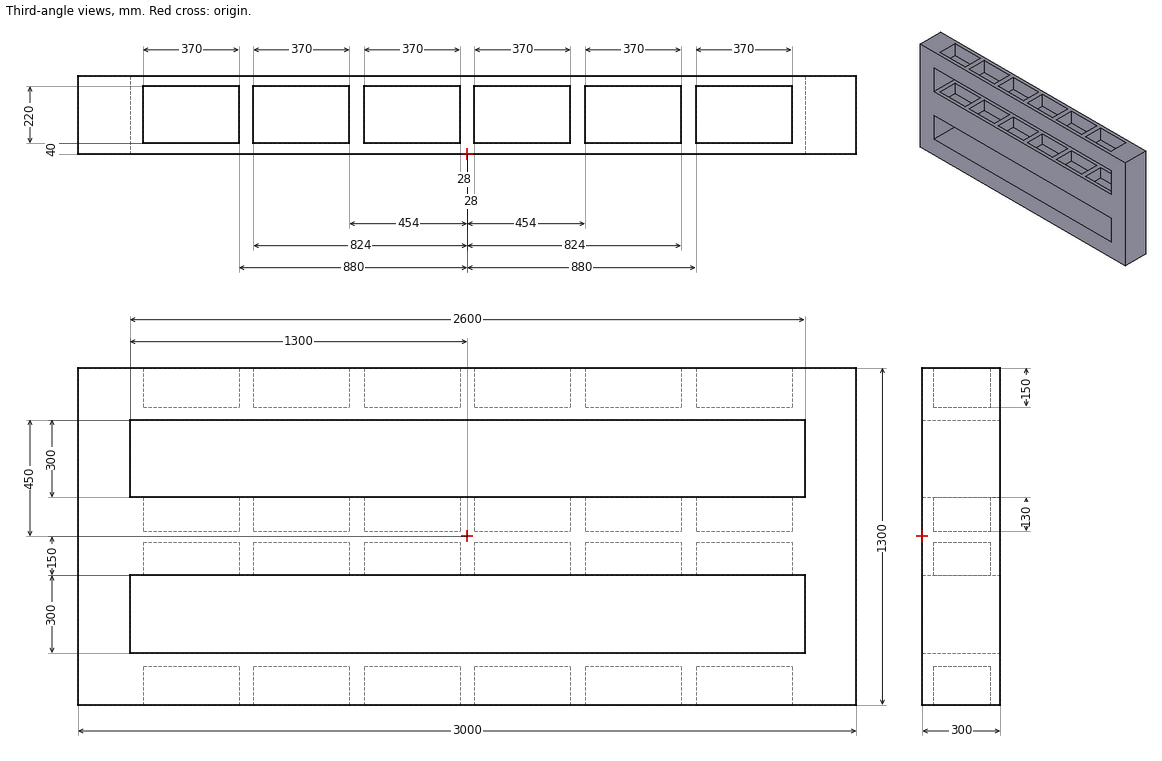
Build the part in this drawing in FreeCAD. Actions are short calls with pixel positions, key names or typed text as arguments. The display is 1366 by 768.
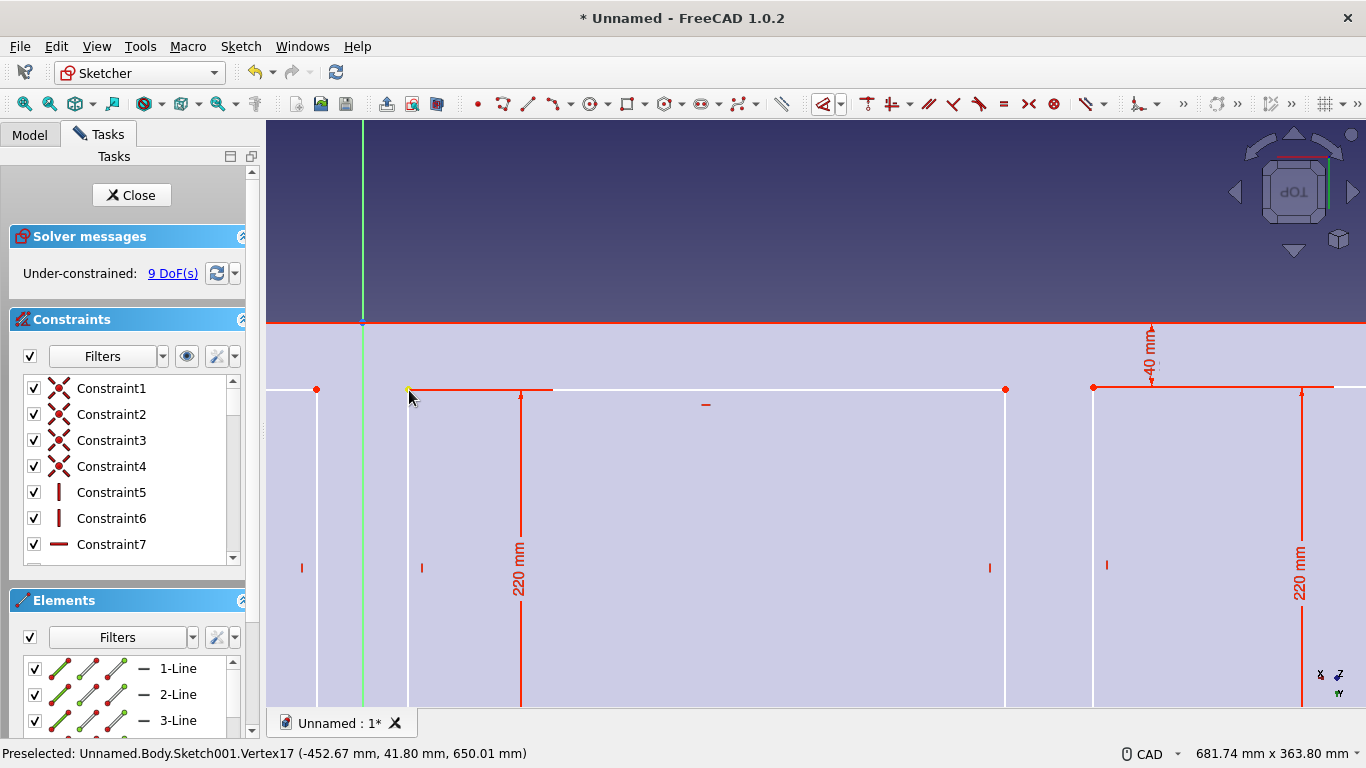
click(408, 390)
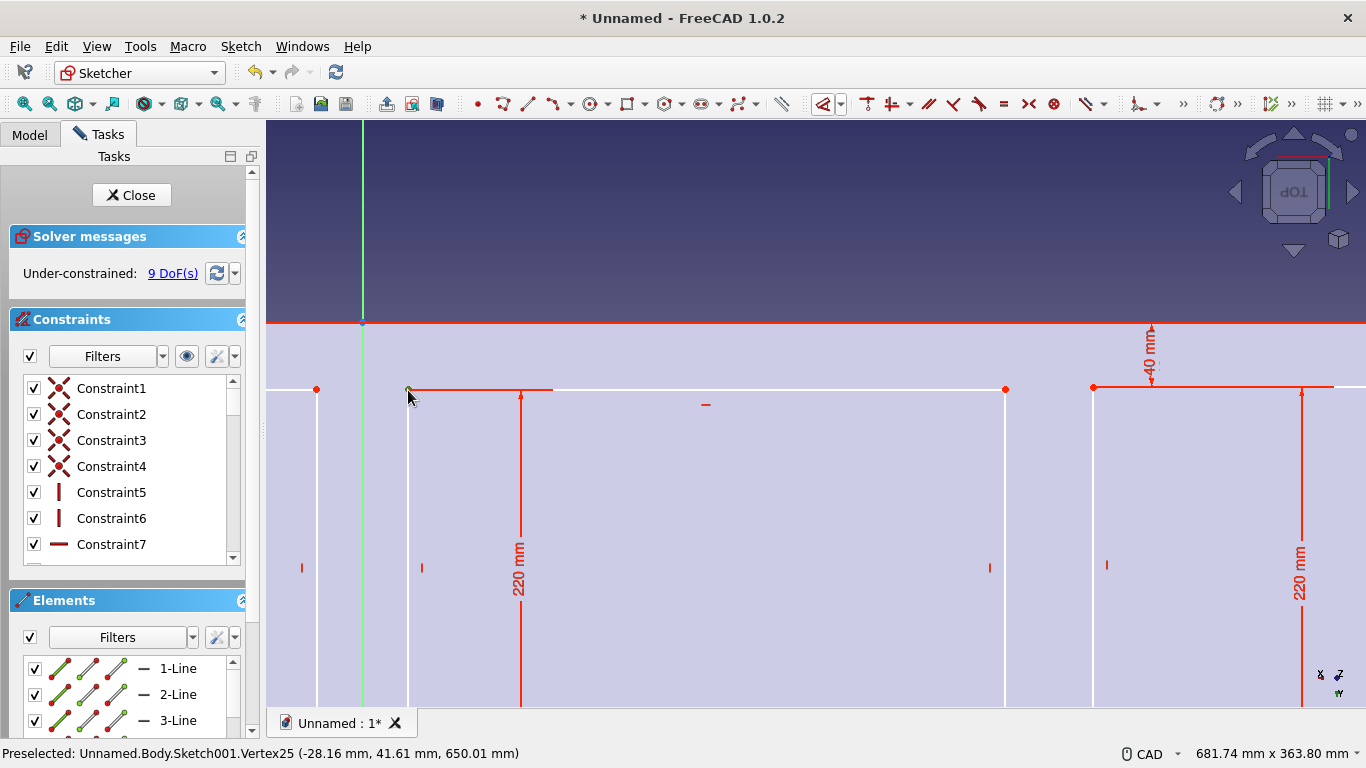
click(840, 104)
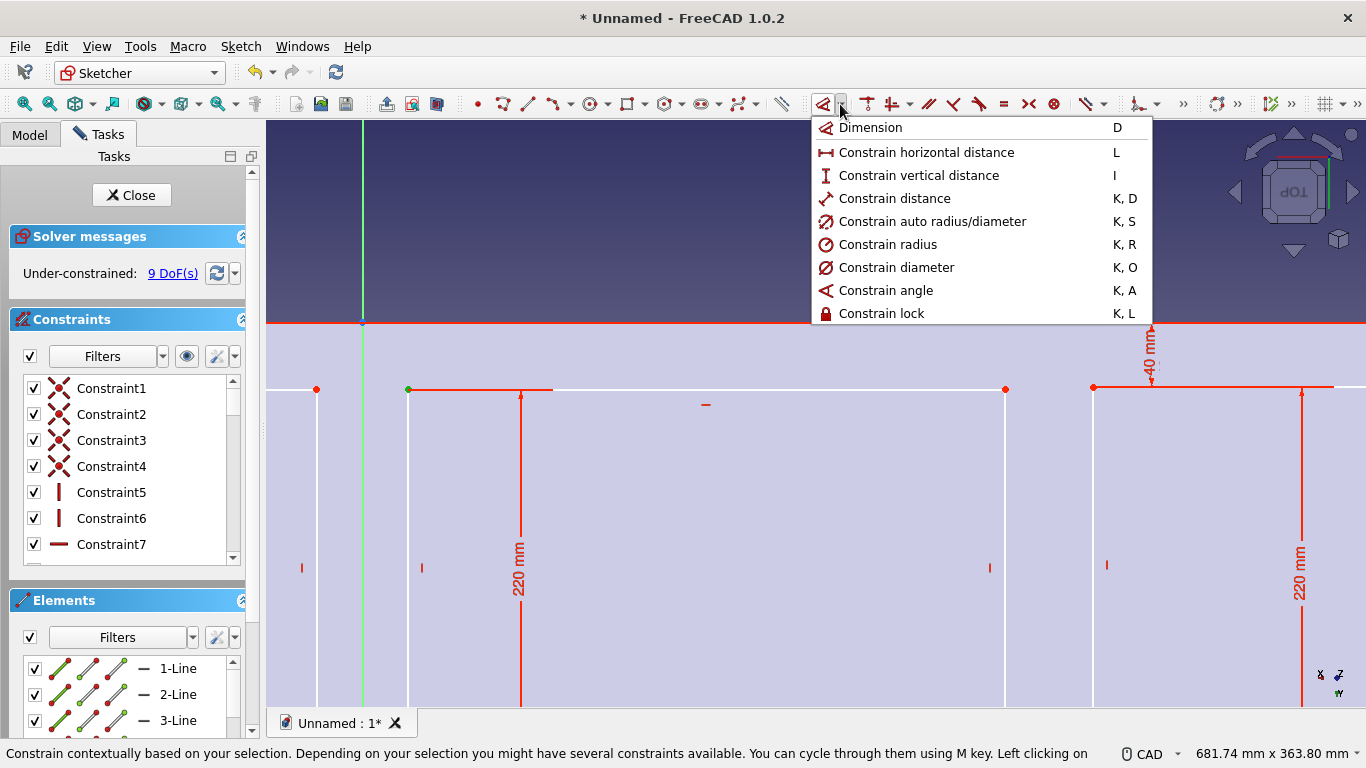
click(982, 152)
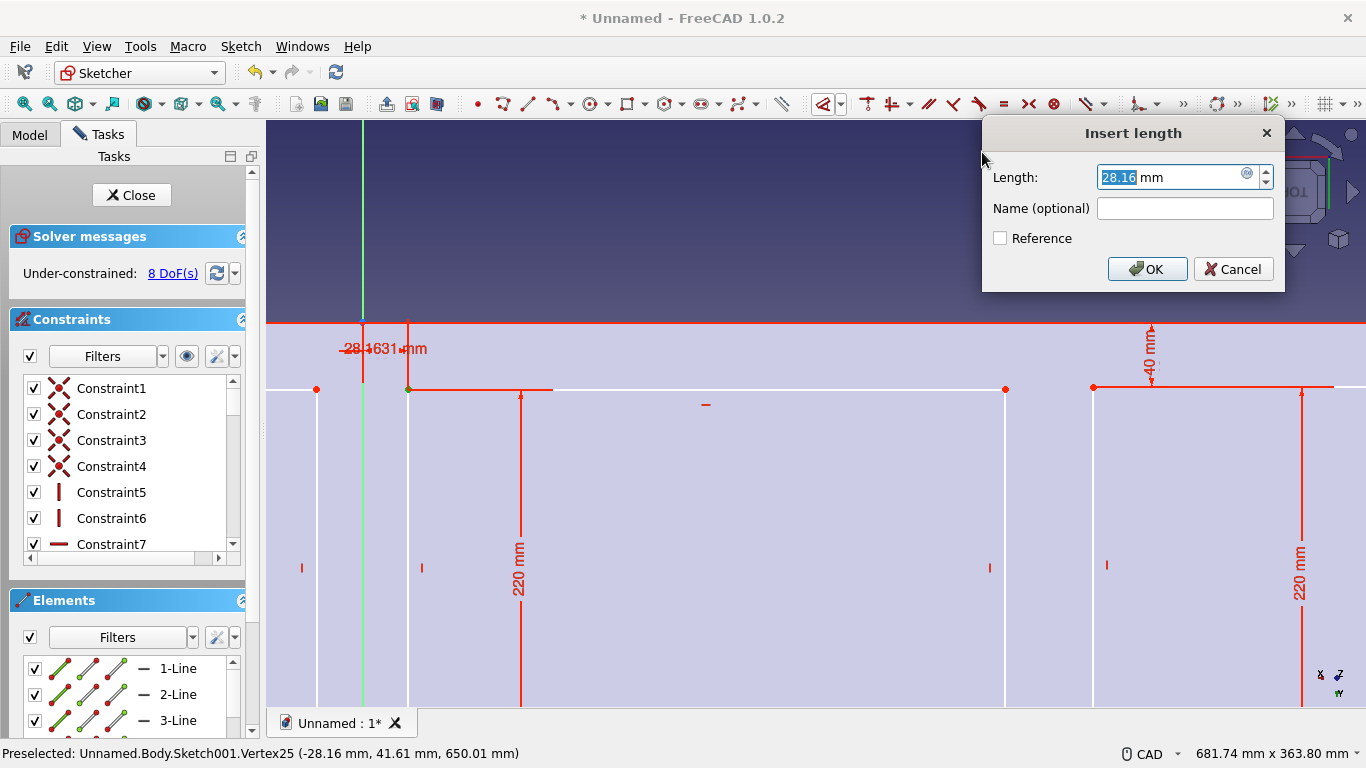
text(28)
key(Return)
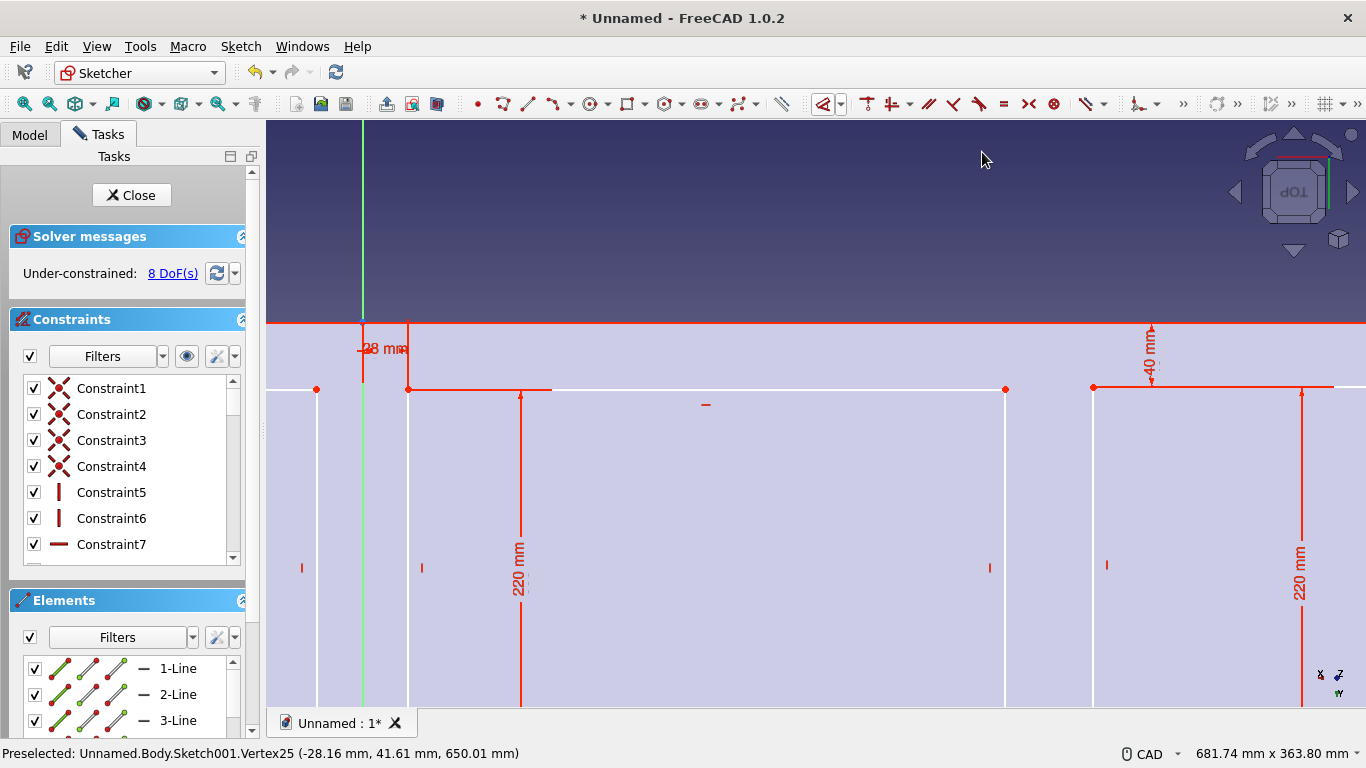
click(408, 390)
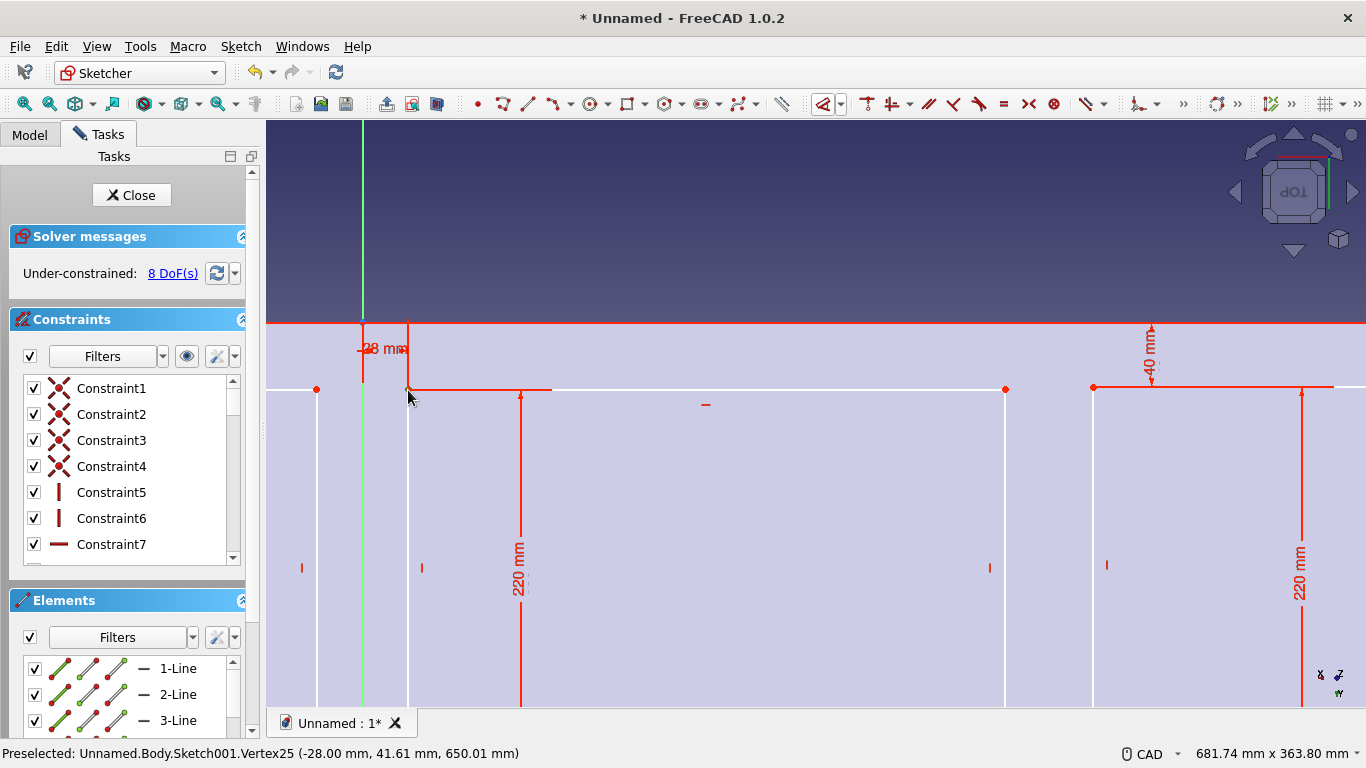
key(i)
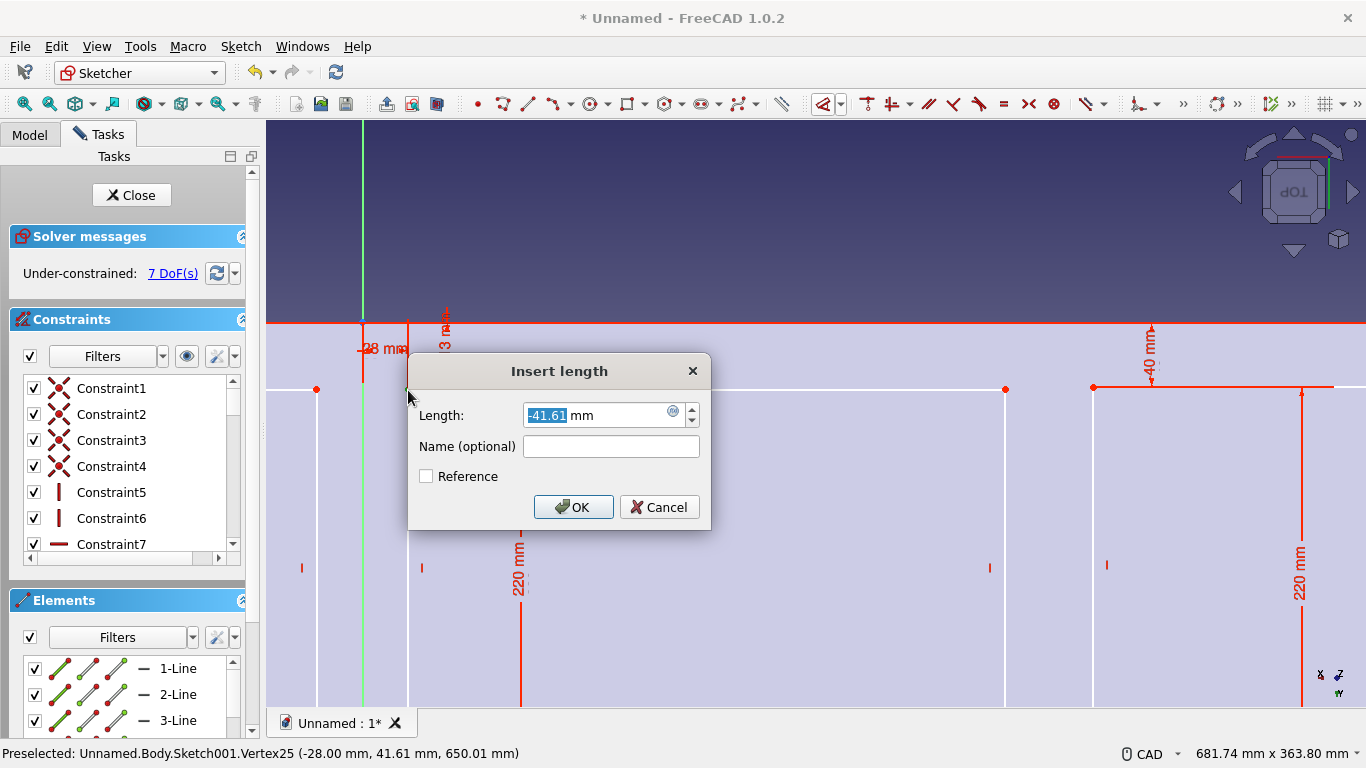
text(-40)
key(Return)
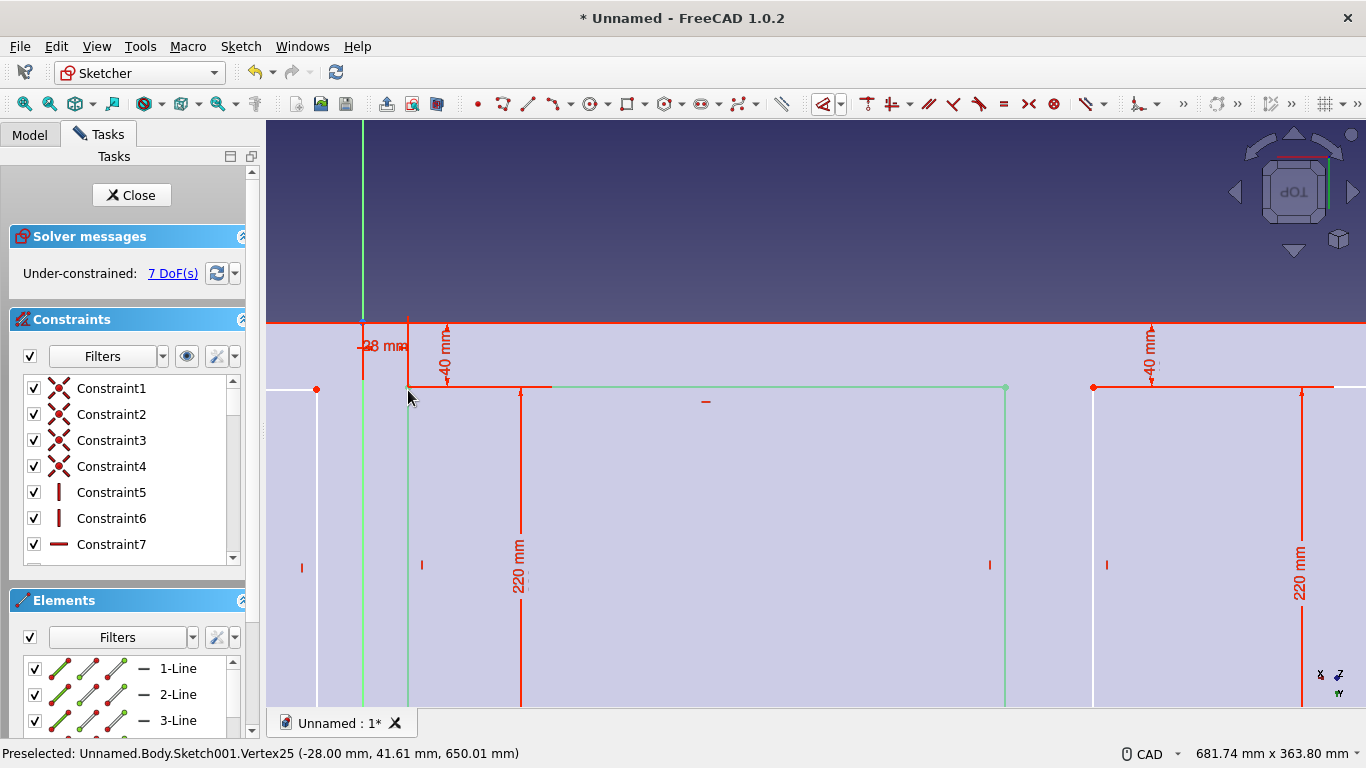
scroll(824, 390, down, 9)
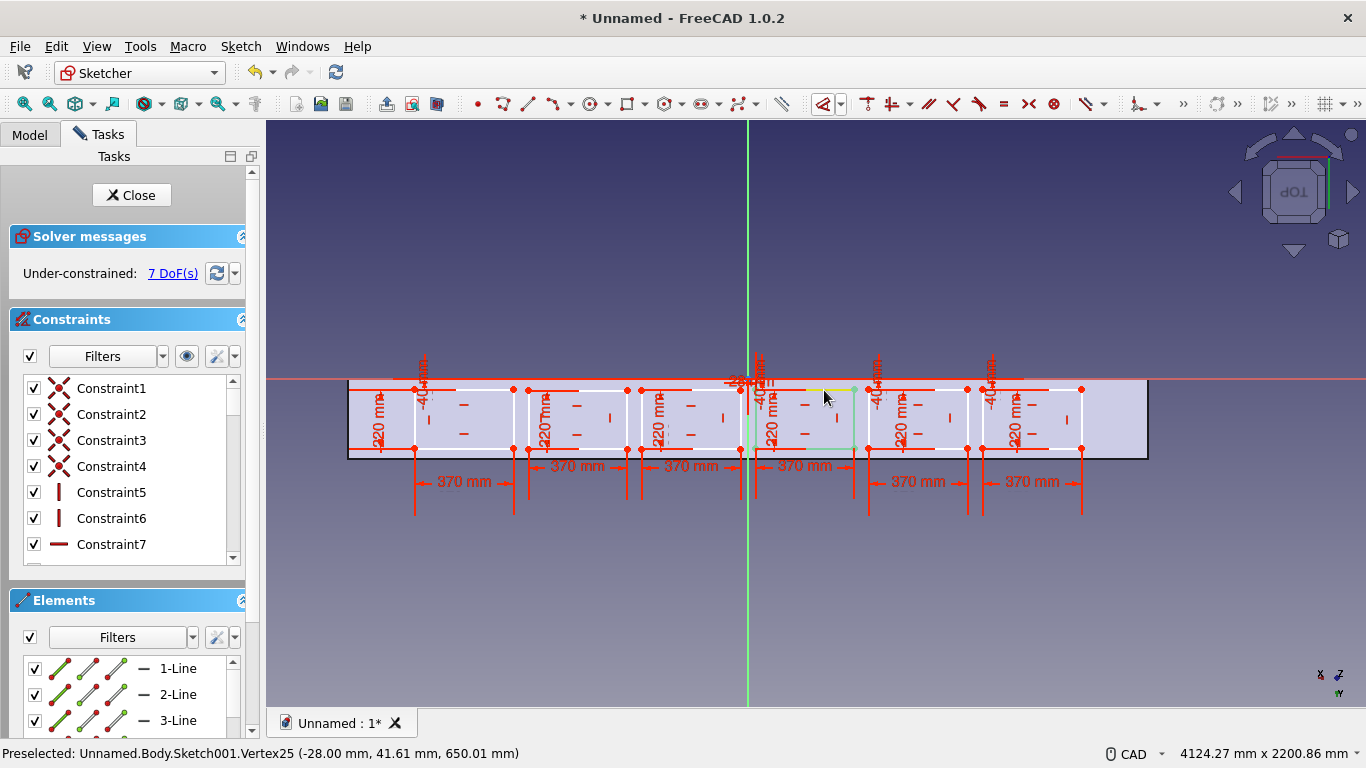
scroll(642, 390, up, 7)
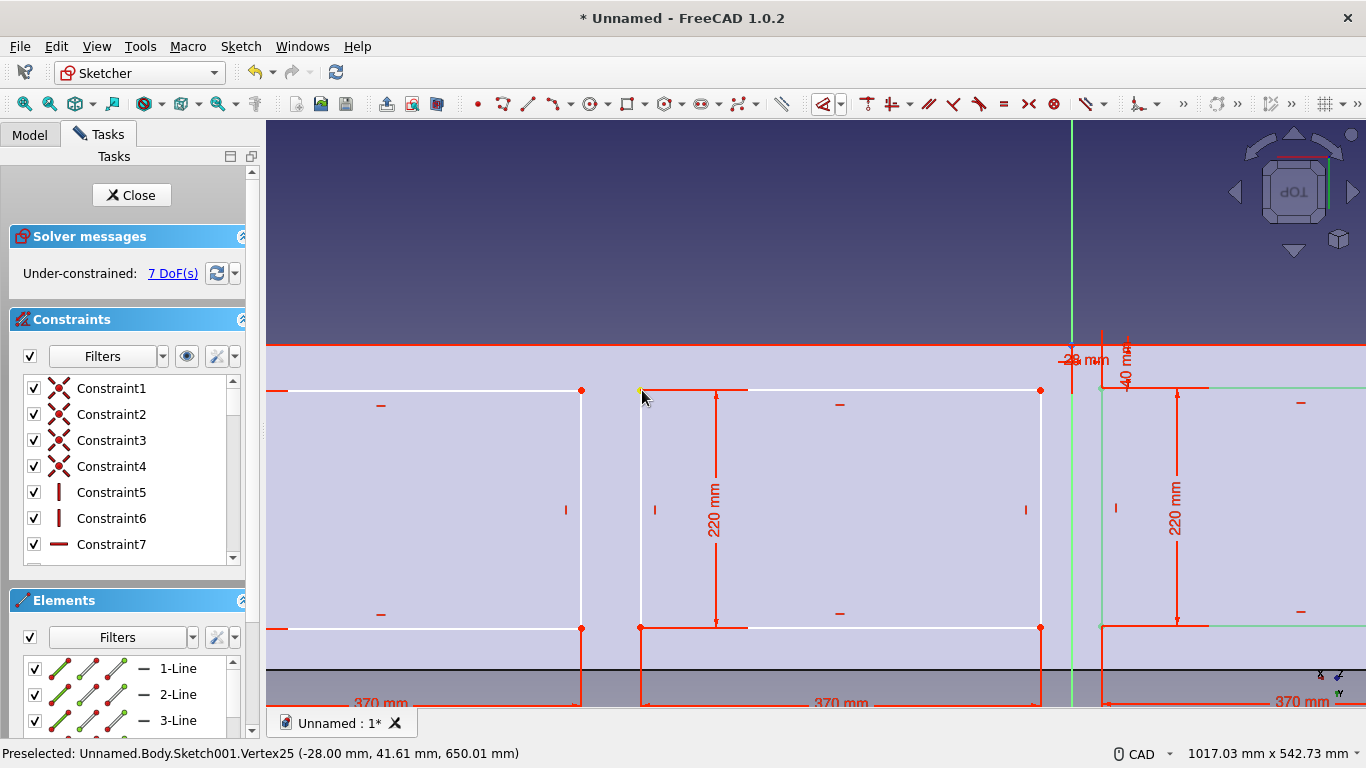
click(641, 390)